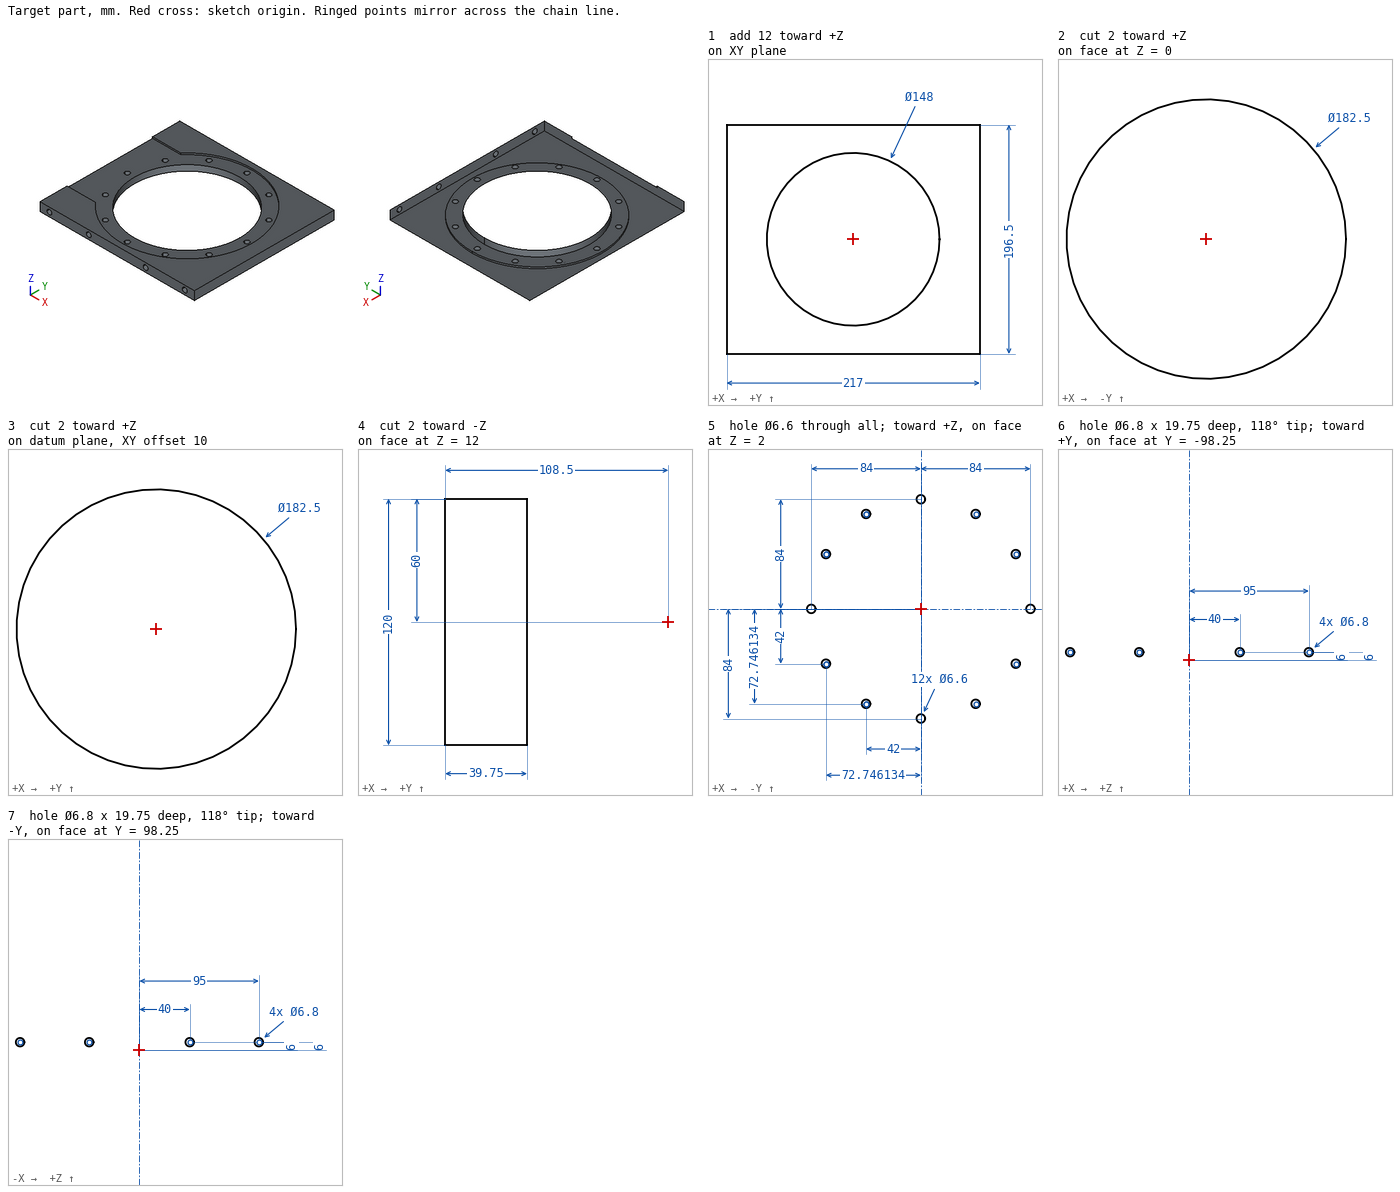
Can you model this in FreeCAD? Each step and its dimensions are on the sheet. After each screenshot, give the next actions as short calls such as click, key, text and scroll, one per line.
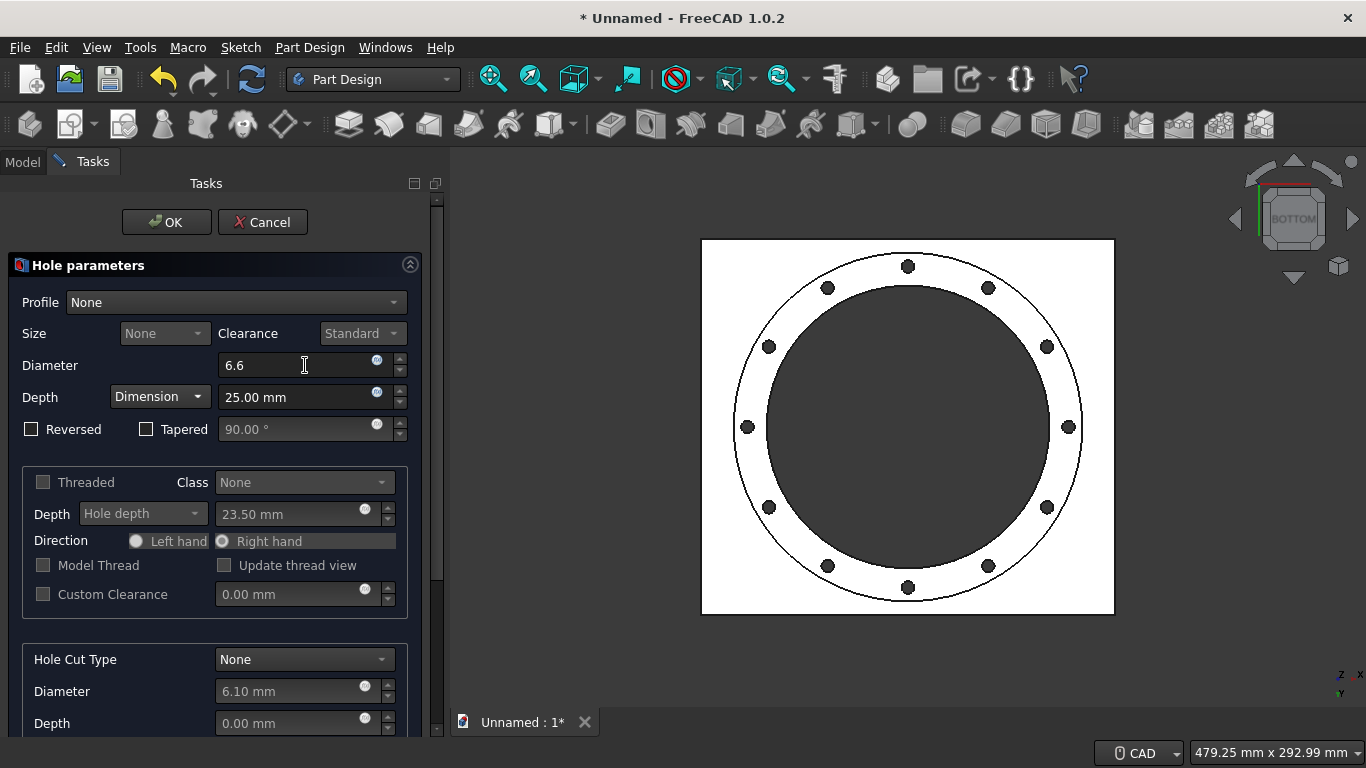
click(161, 396)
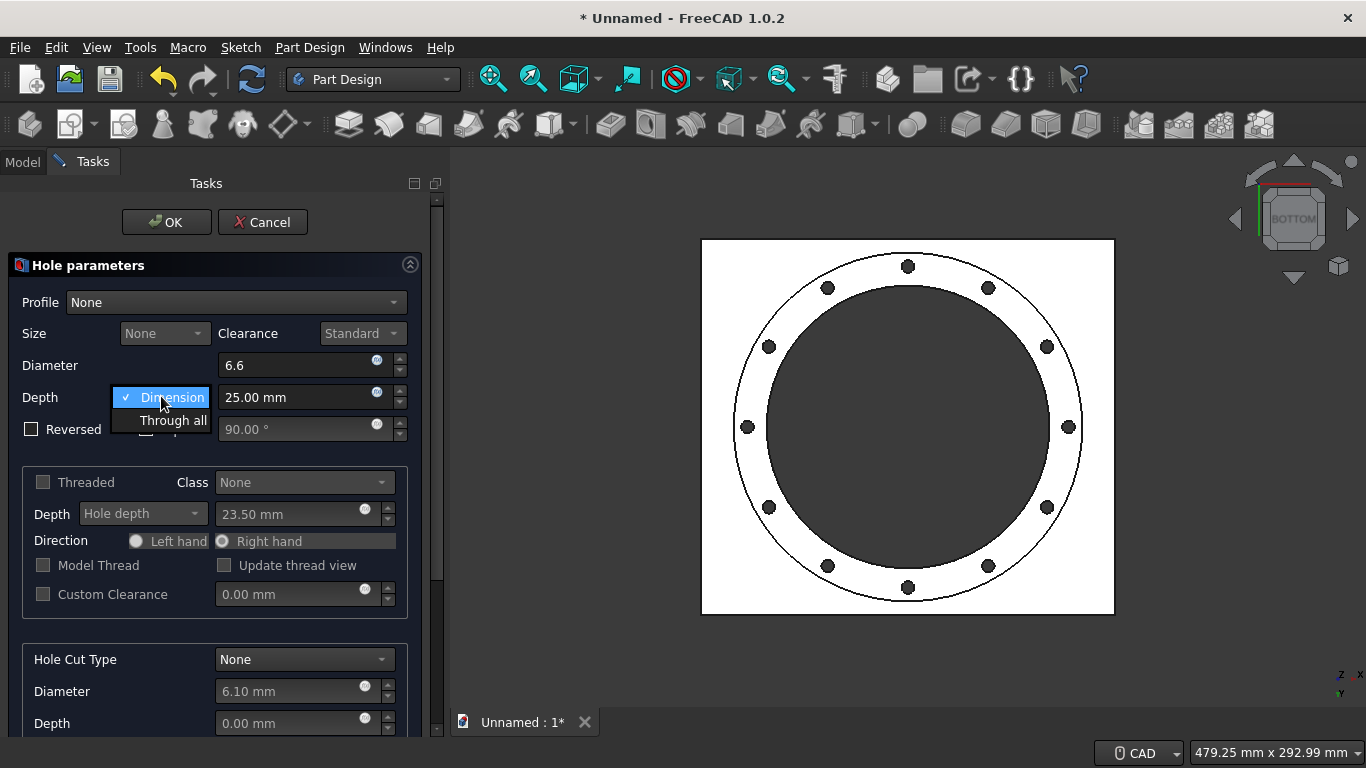
click(160, 420)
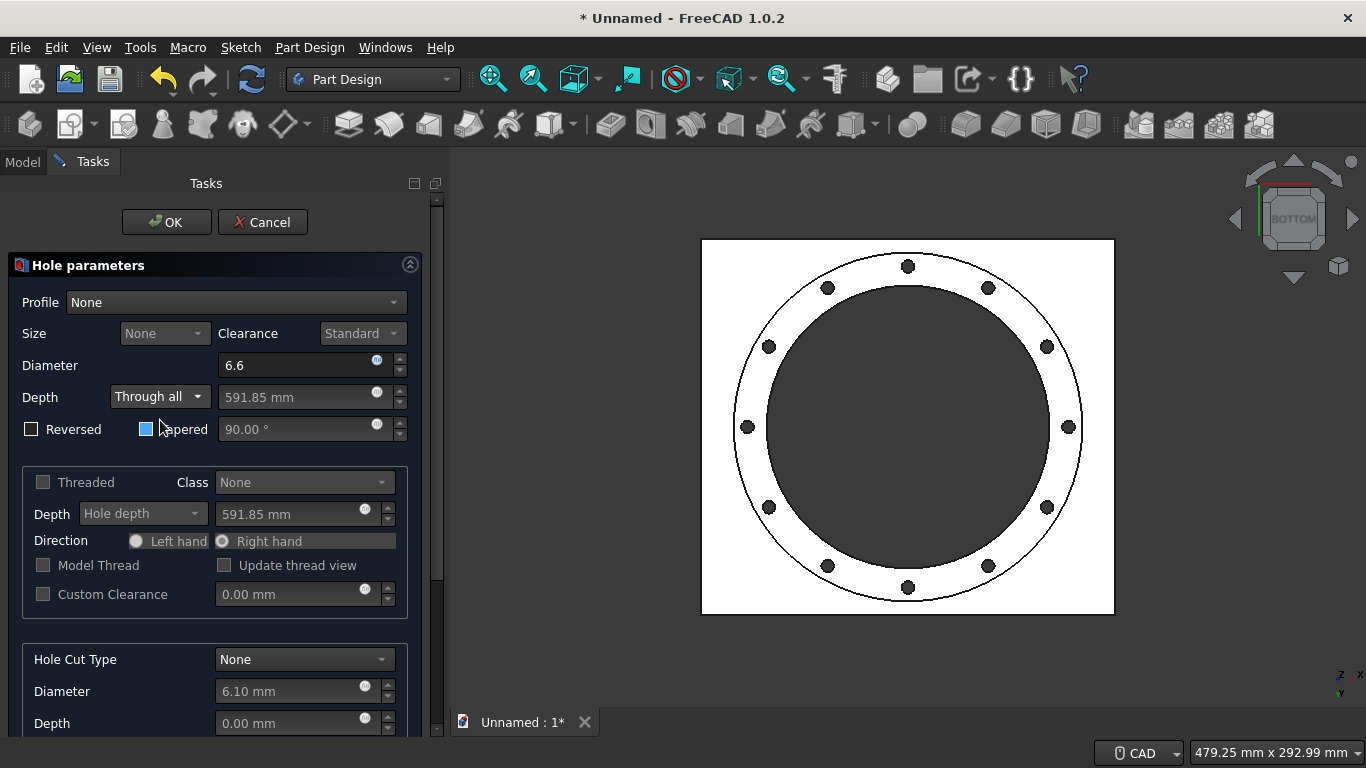
click(167, 222)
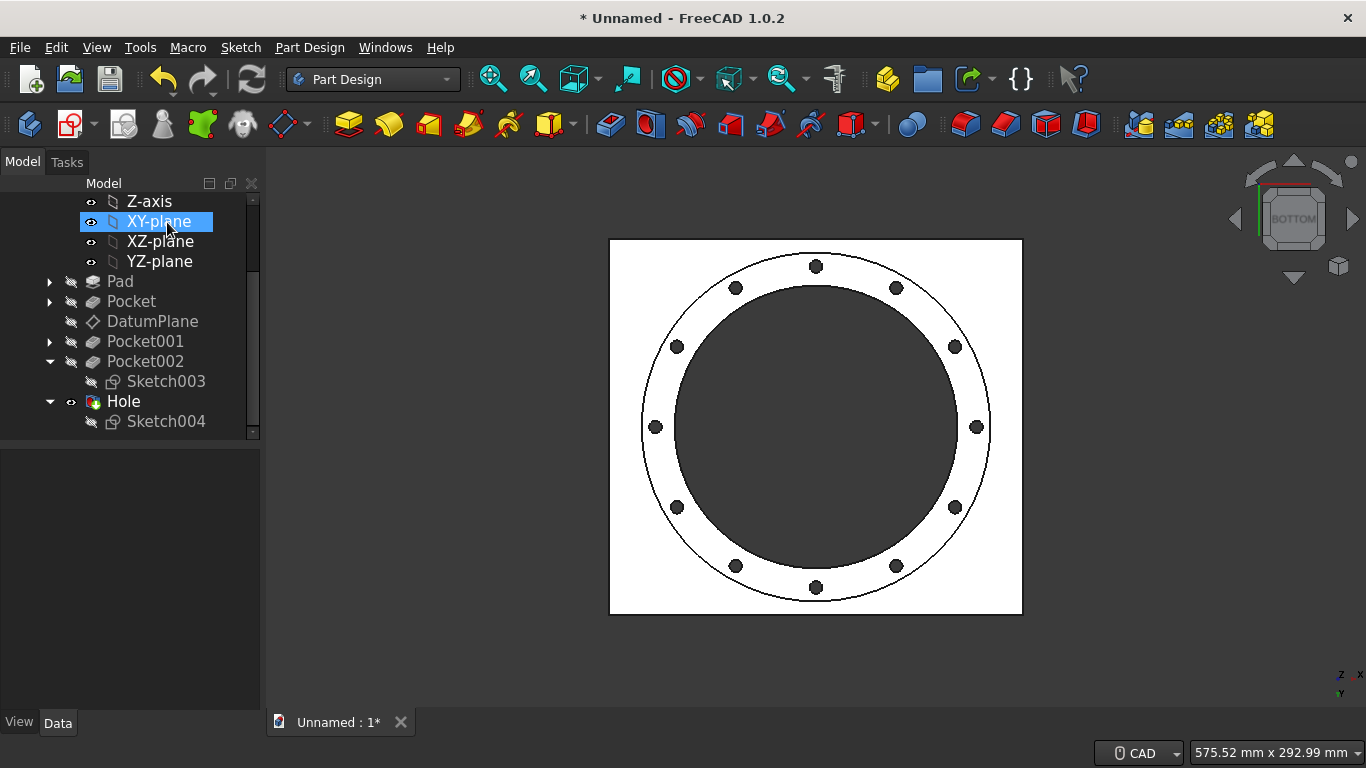
key(0)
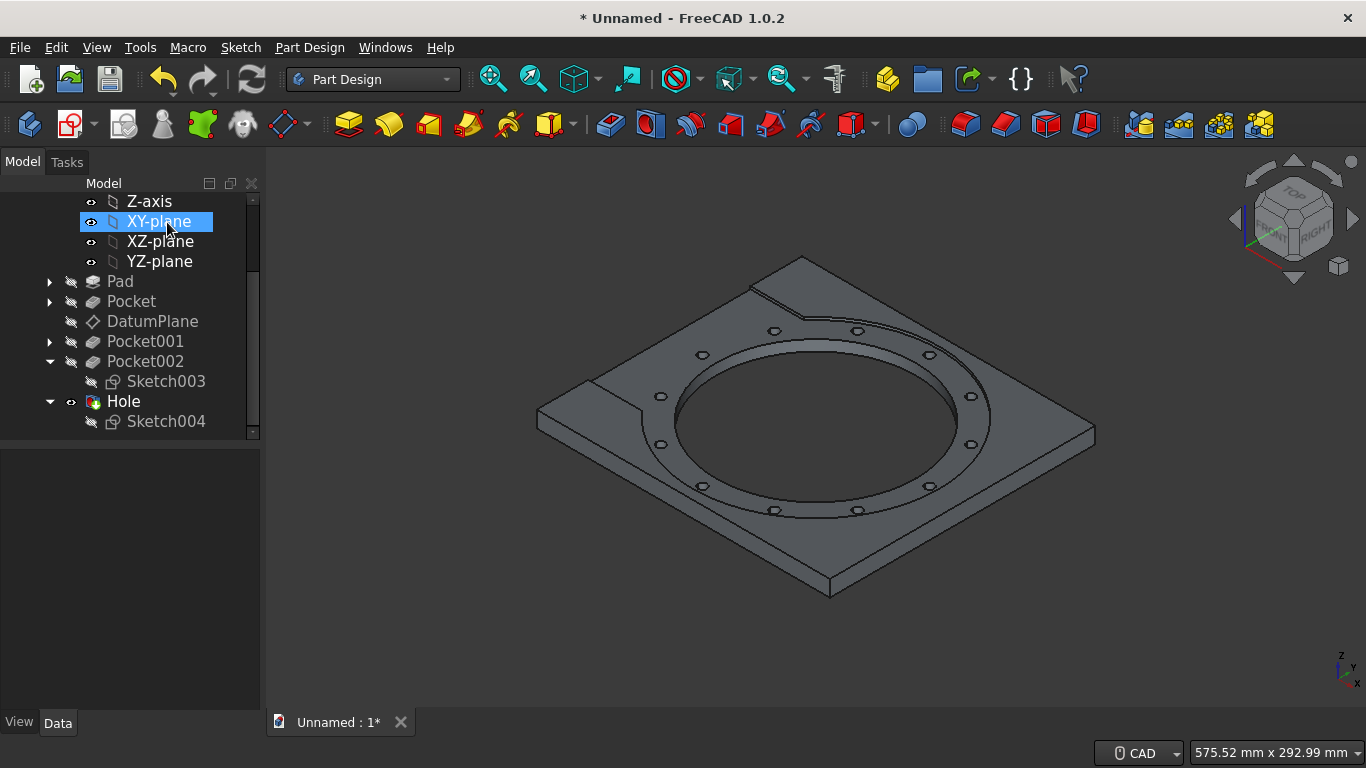
key(1)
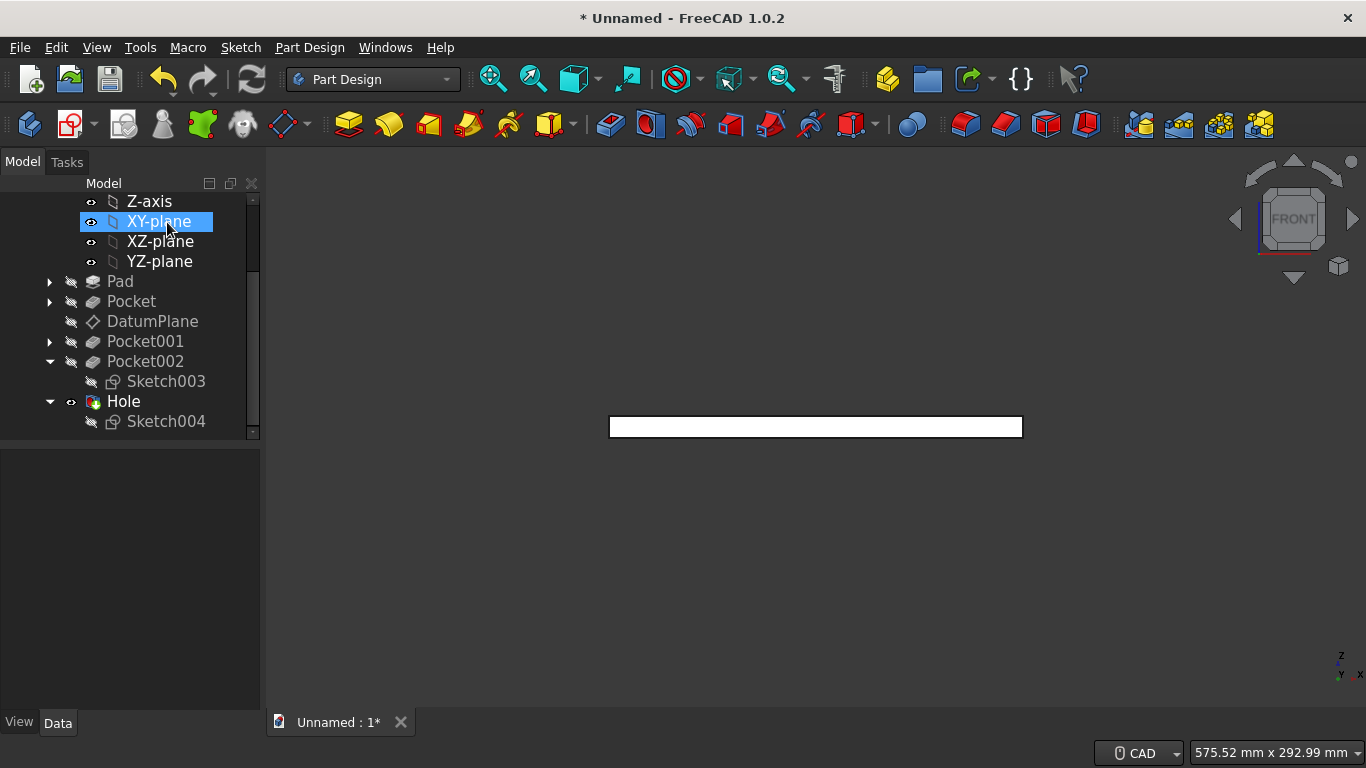
click(494, 80)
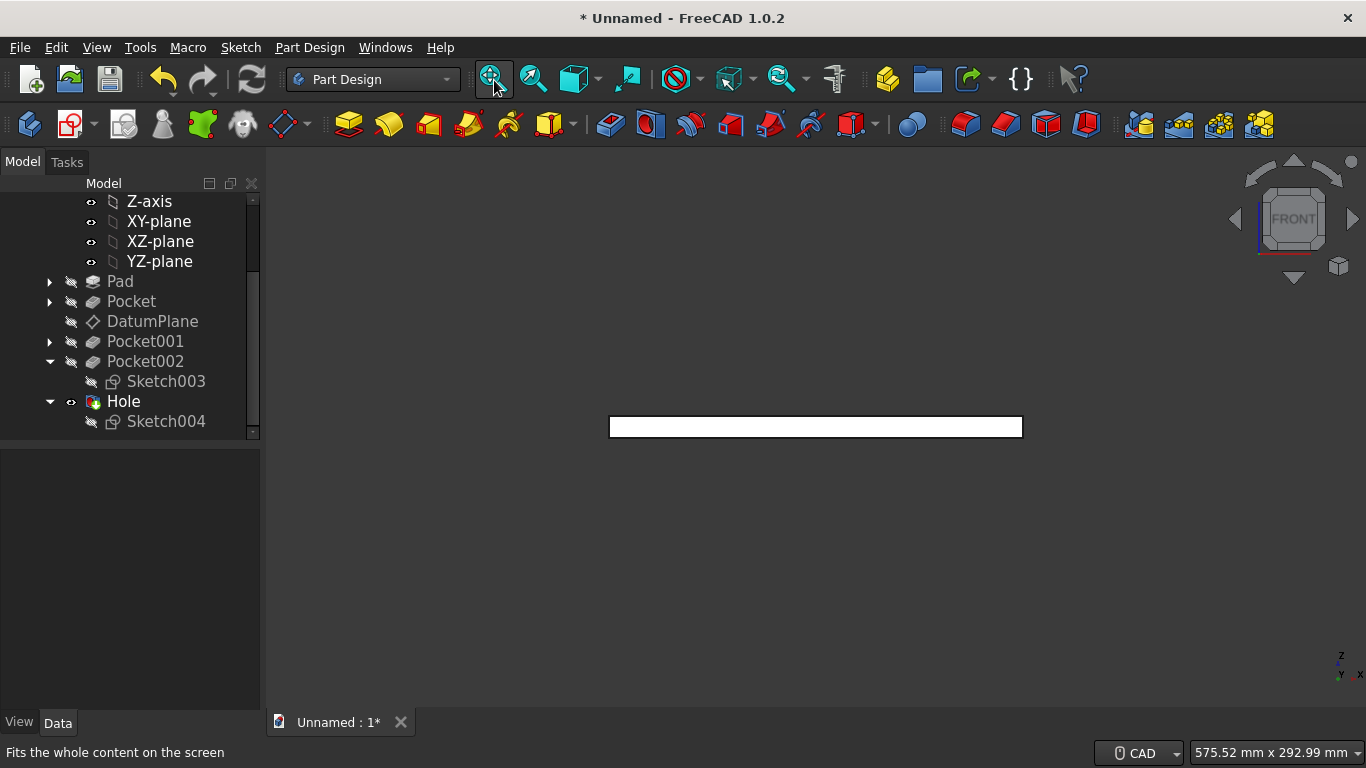
click(994, 426)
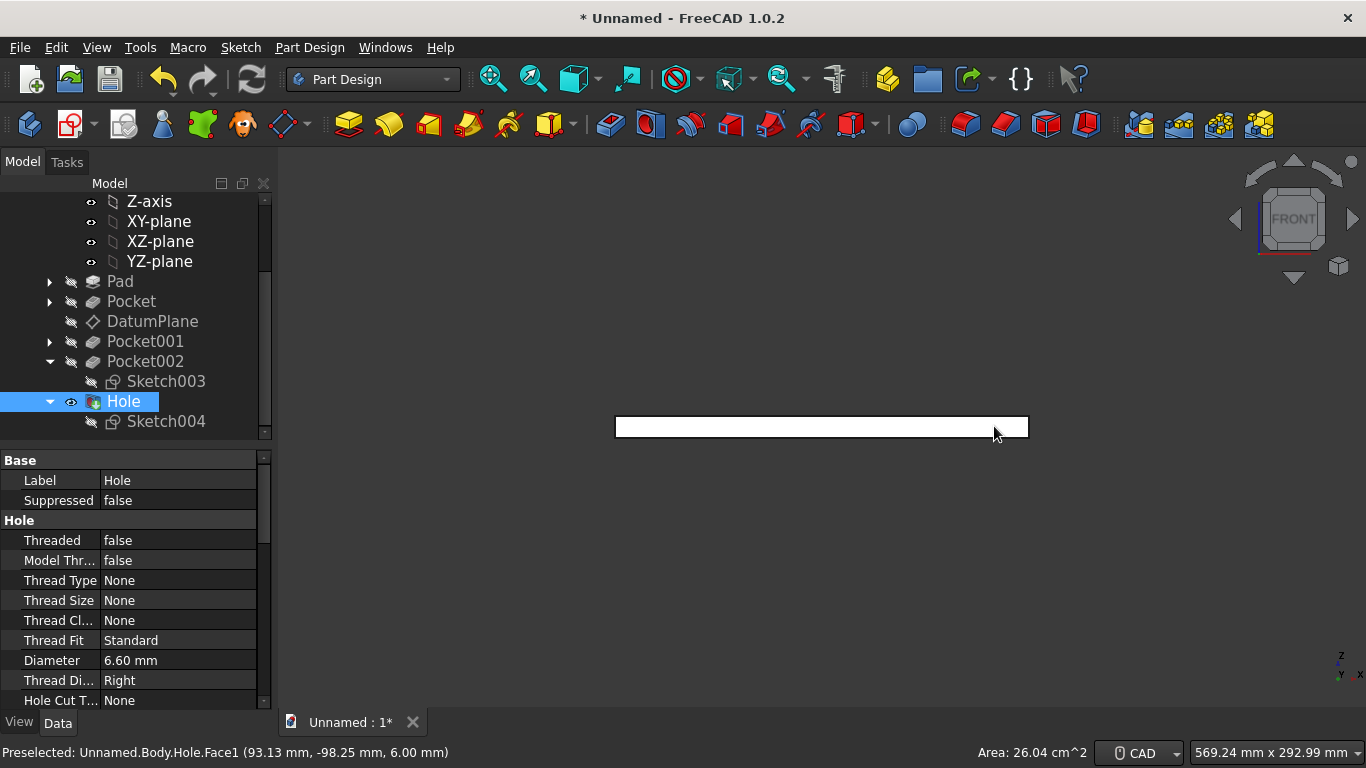
click(70, 124)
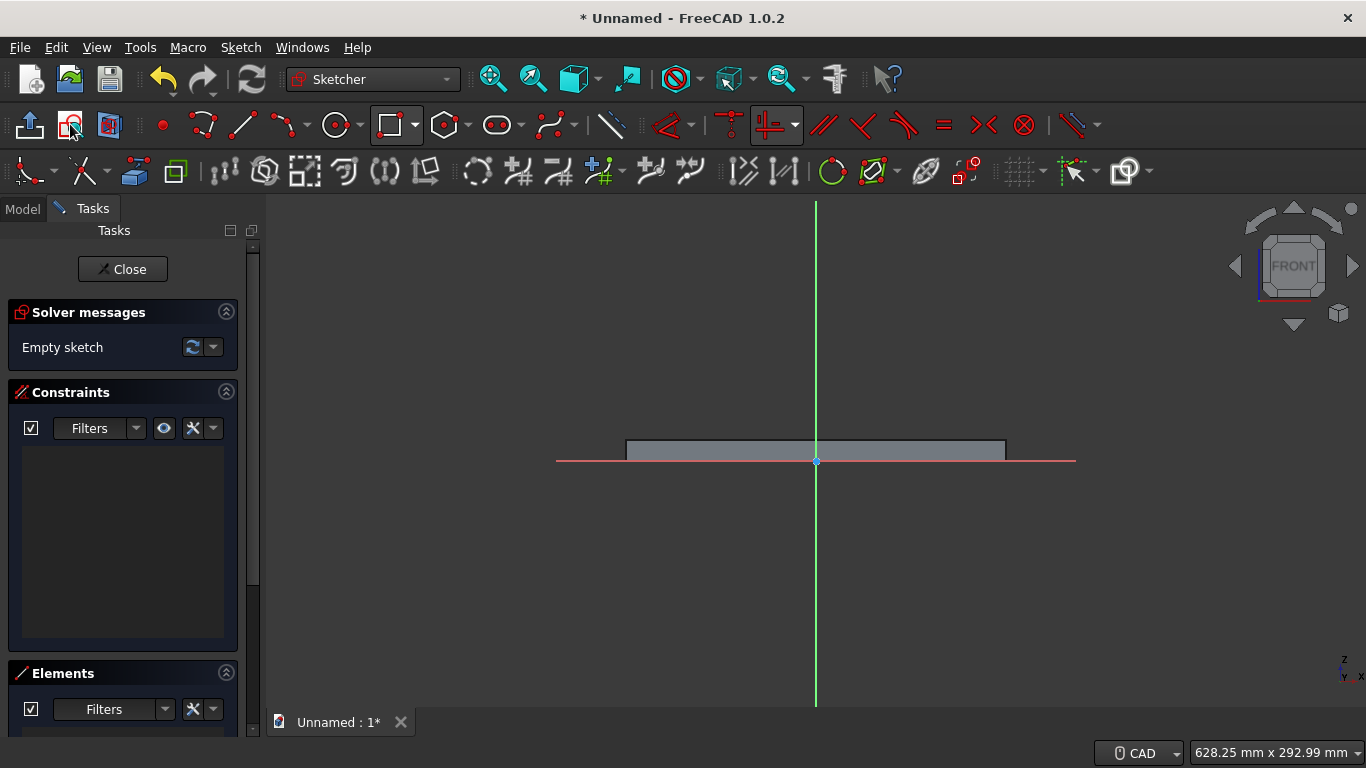
scroll(899, 456, up, 3)